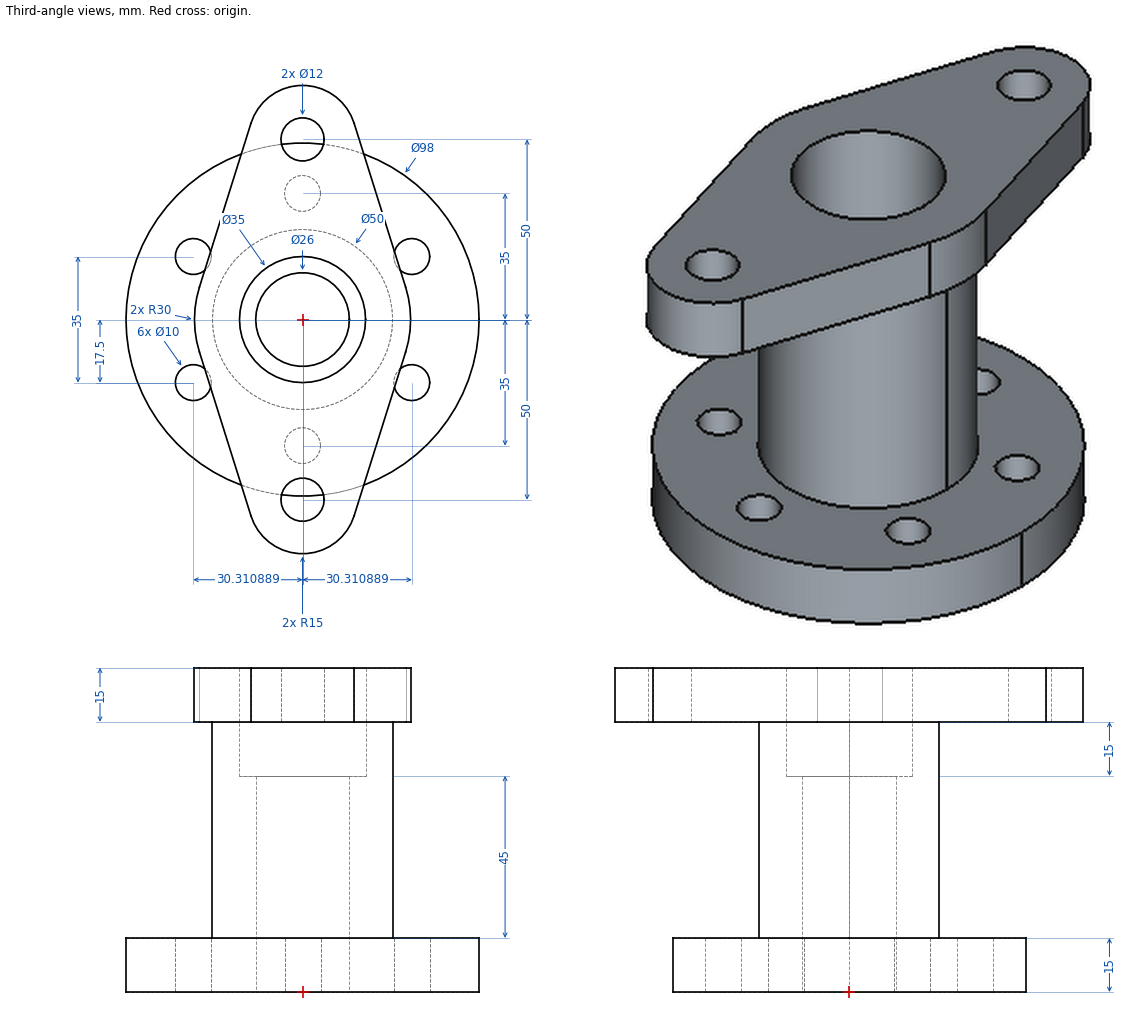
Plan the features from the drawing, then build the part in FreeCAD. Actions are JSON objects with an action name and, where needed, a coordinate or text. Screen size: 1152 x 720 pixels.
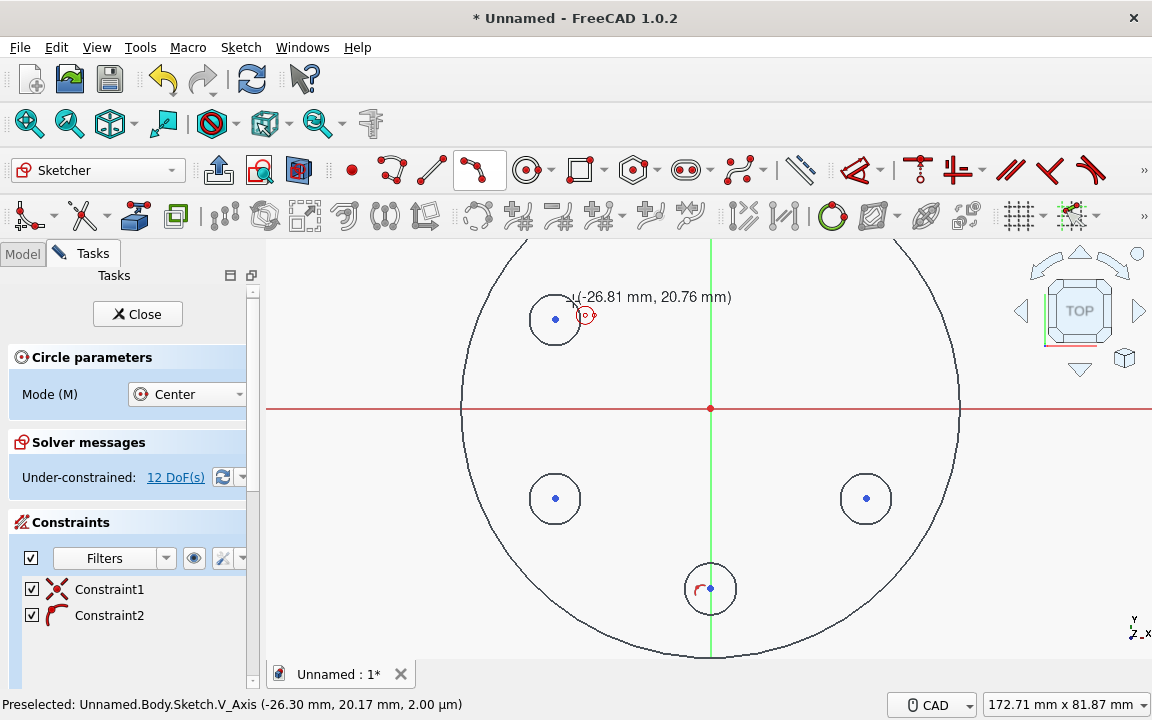
{"action": "left_click", "coordinate": [711, 409]}
{"action": "left_click", "coordinate": [758, 361]}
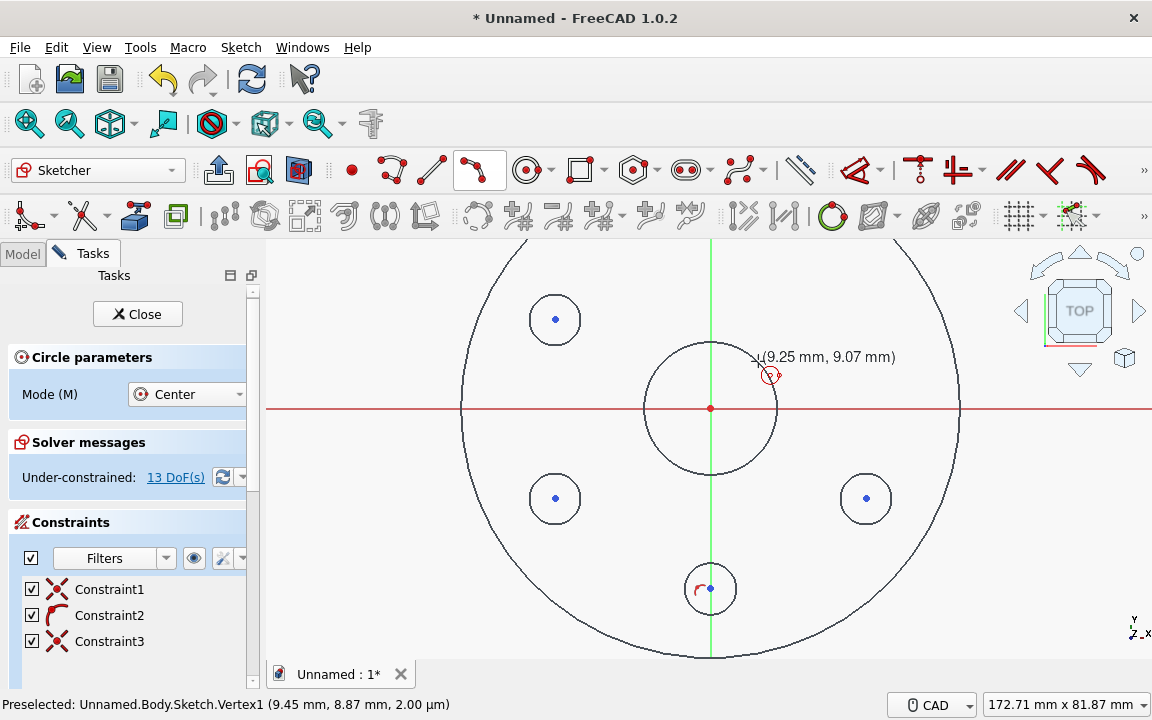
{"action": "left_click", "coordinate": [866, 319]}
{"action": "left_click", "coordinate": [884, 301]}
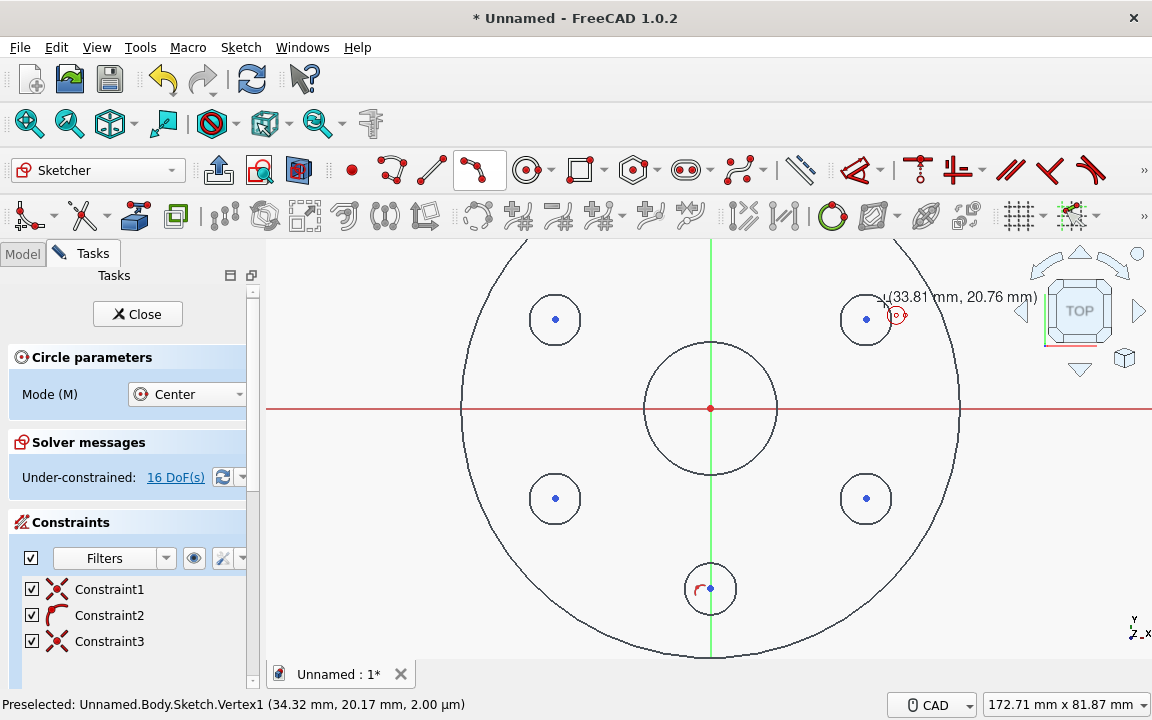
{"action": "scroll", "coordinate": [555, 498], "scroll_direction": "down", "scroll_amount": 3}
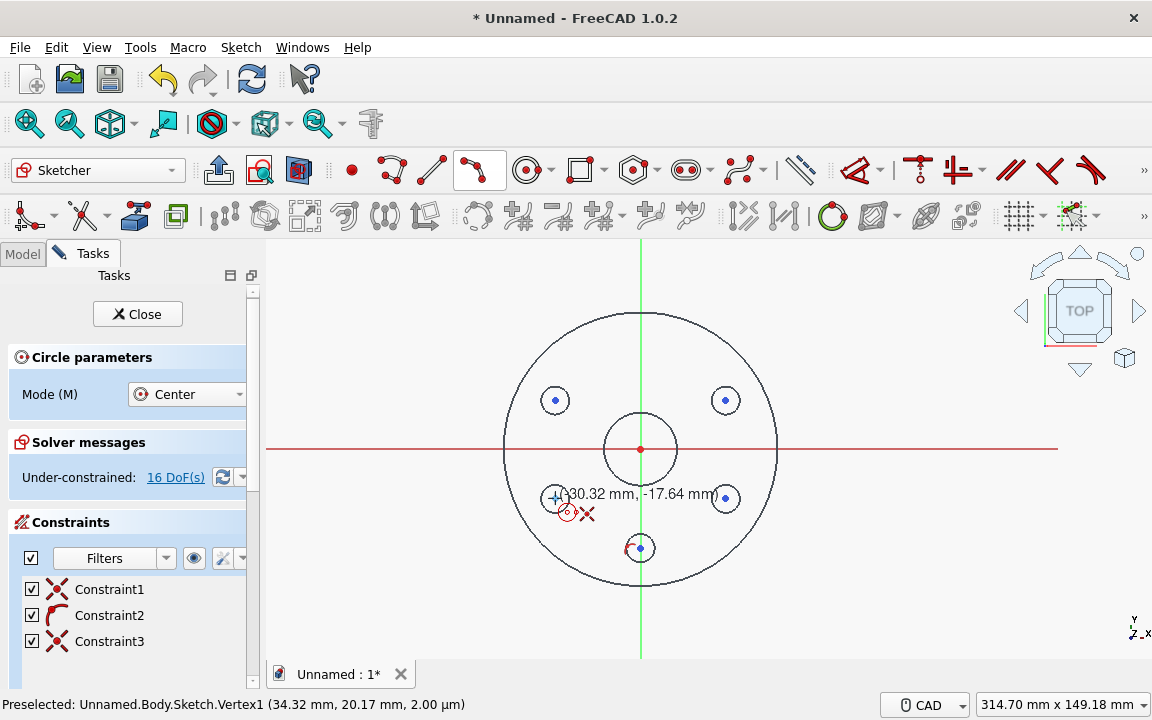
{"action": "scroll", "coordinate": [641, 351], "scroll_direction": "up", "scroll_amount": 3}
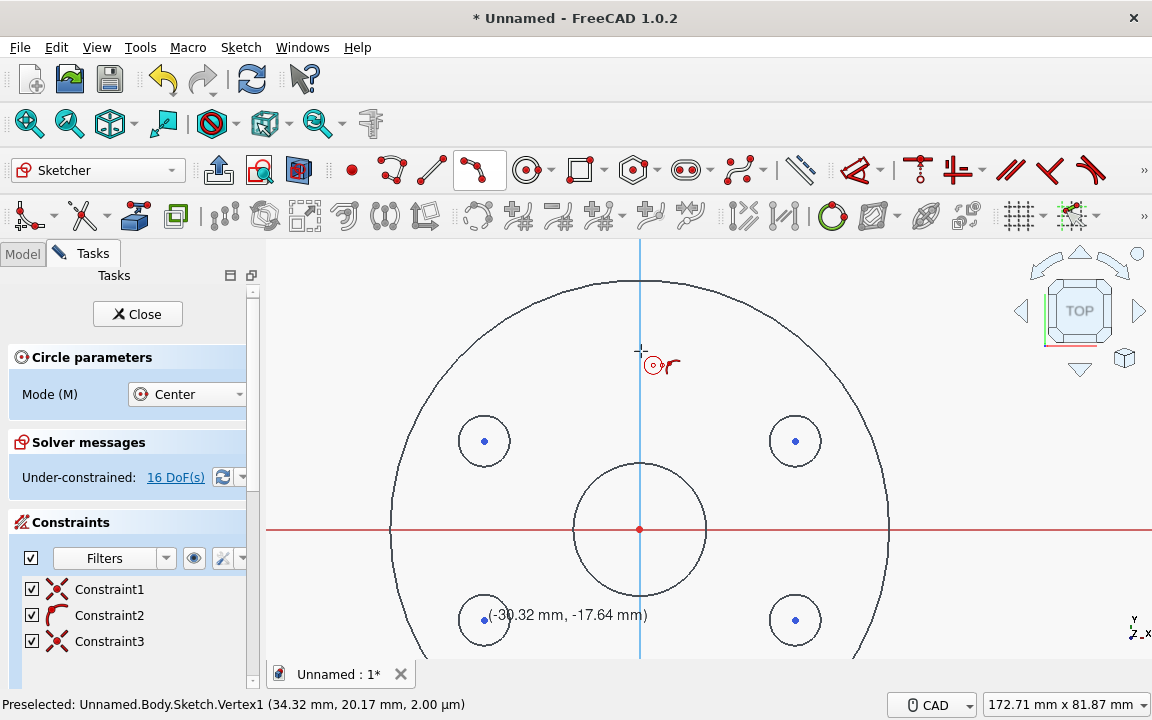
{"action": "left_click", "coordinate": [640, 350]}
{"action": "left_click", "coordinate": [658, 332]}
{"action": "key", "text": "Escape"}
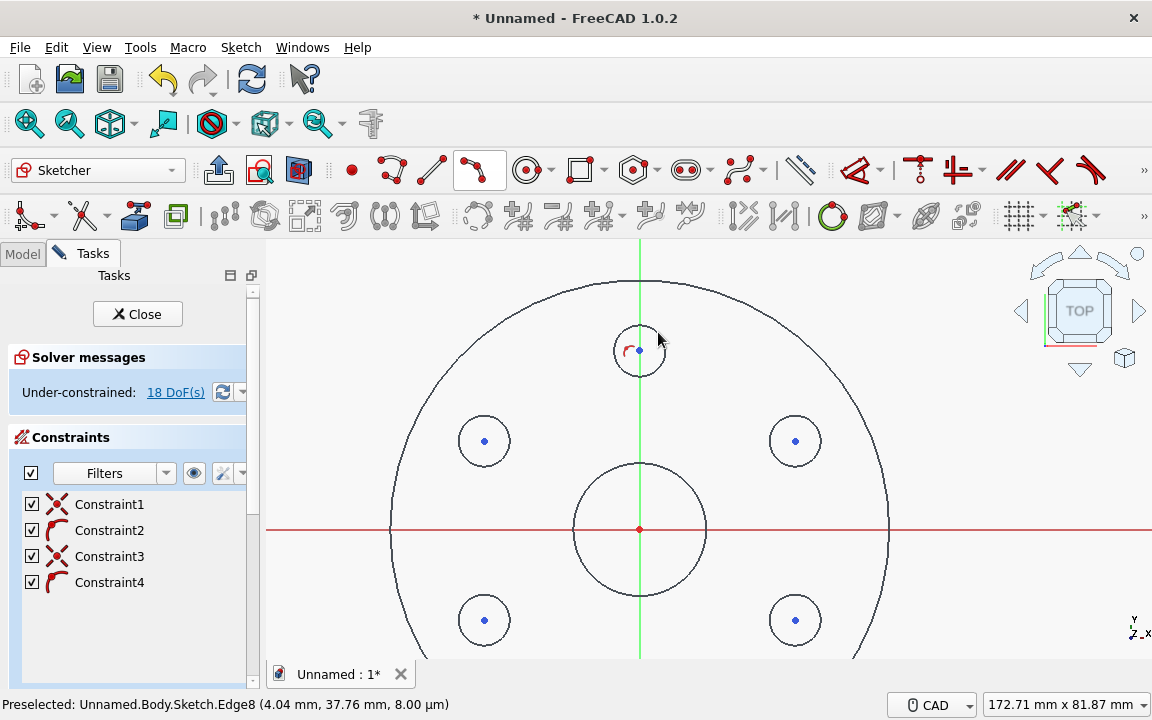
{"action": "left_click", "coordinate": [502, 602]}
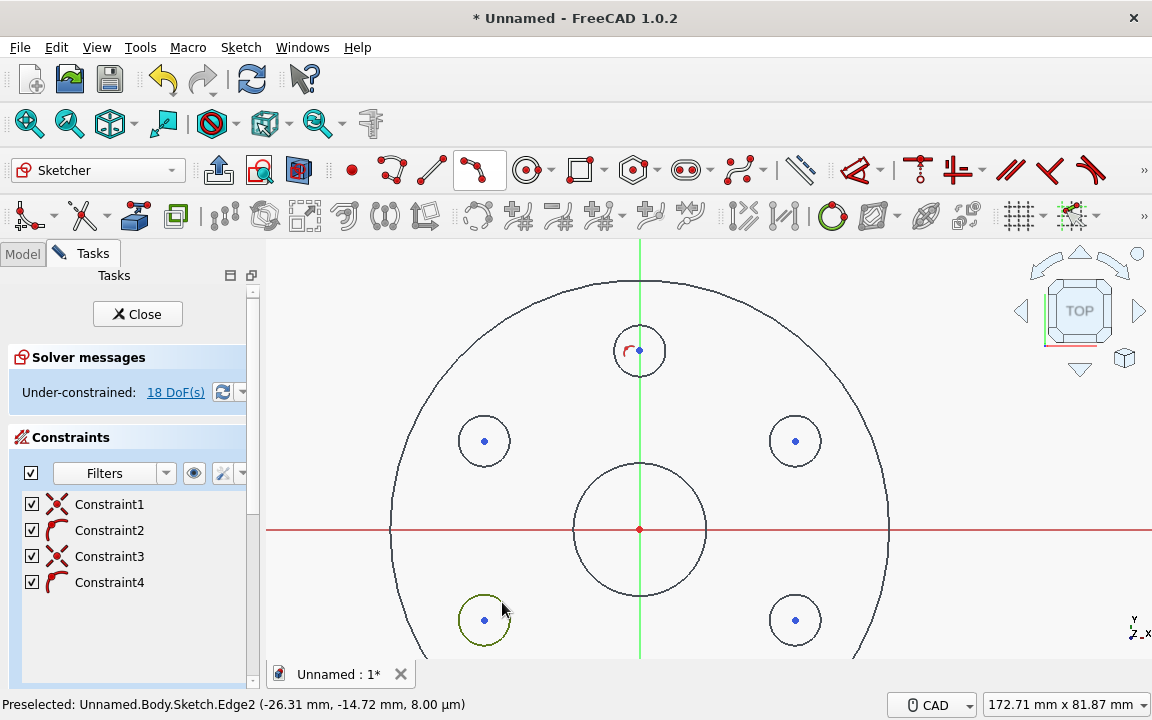
{"action": "scroll", "coordinate": [641, 351], "scroll_direction": "down", "scroll_amount": 3}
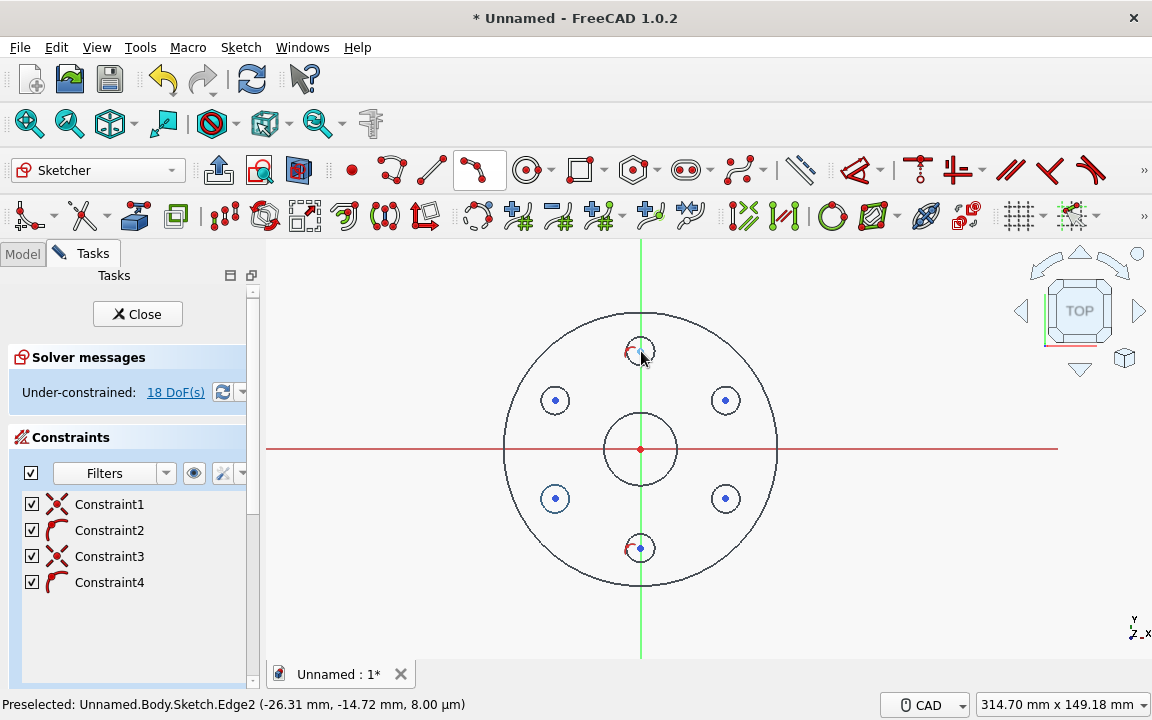
{"action": "scroll", "coordinate": [650, 538], "scroll_direction": "up", "scroll_amount": 2}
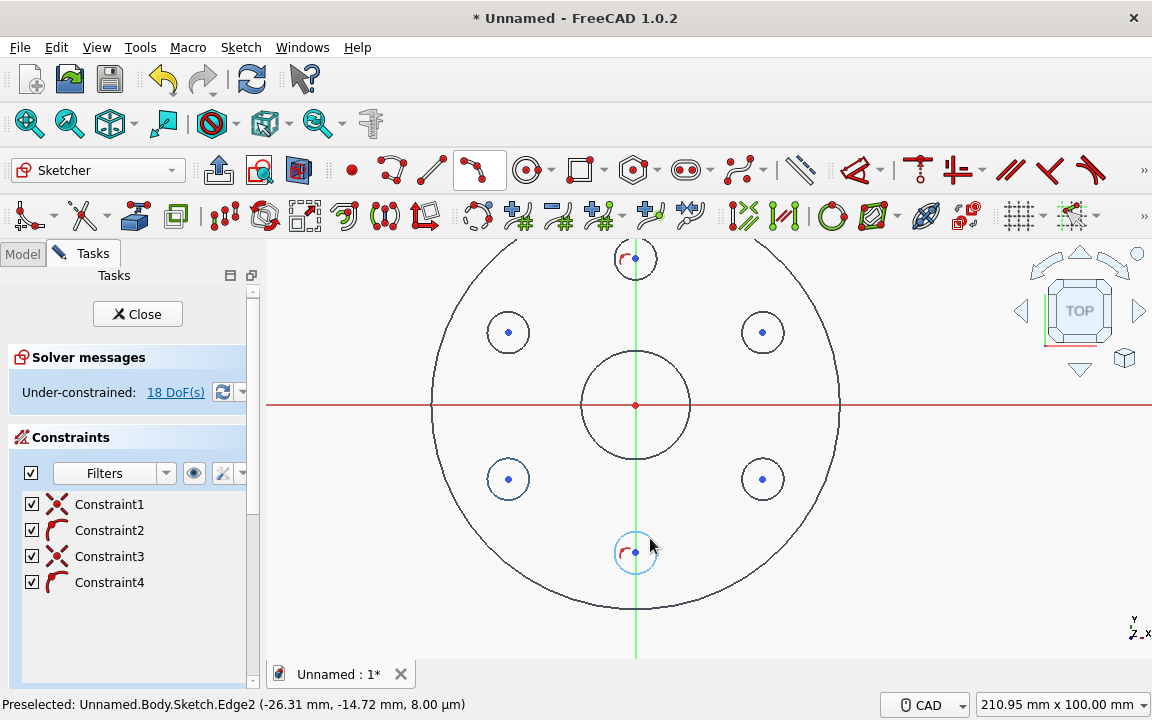
{"action": "left_click", "coordinate": [651, 538]}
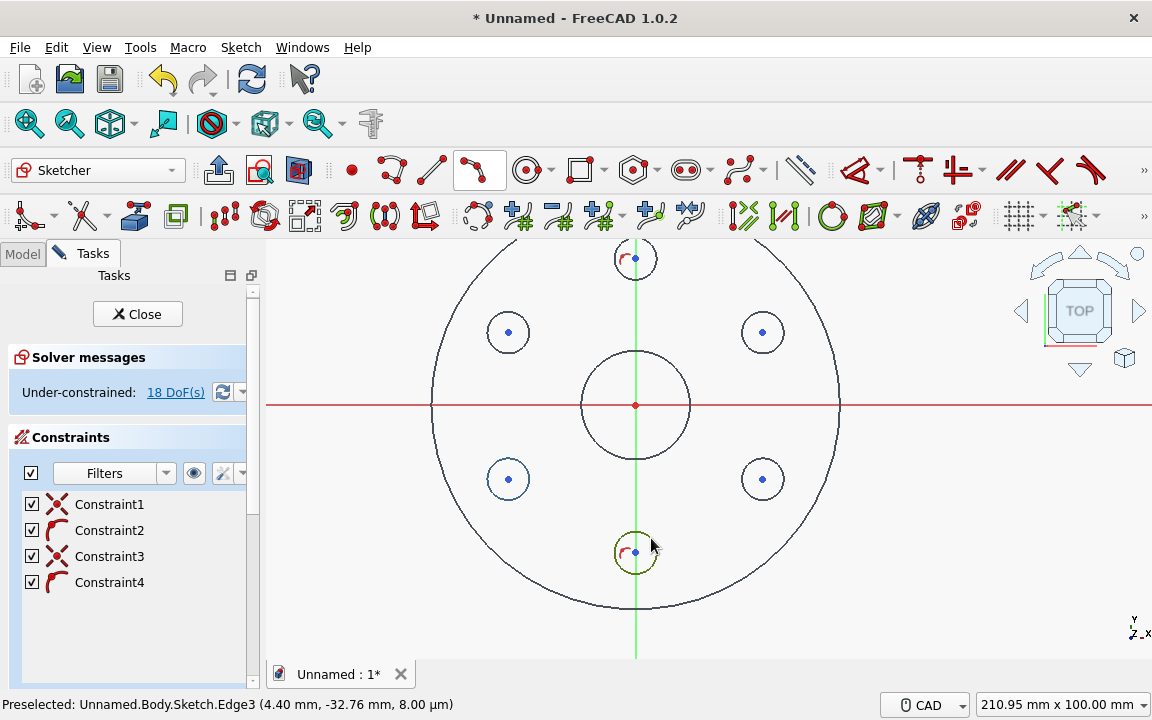
{"action": "left_click", "coordinate": [778, 464]}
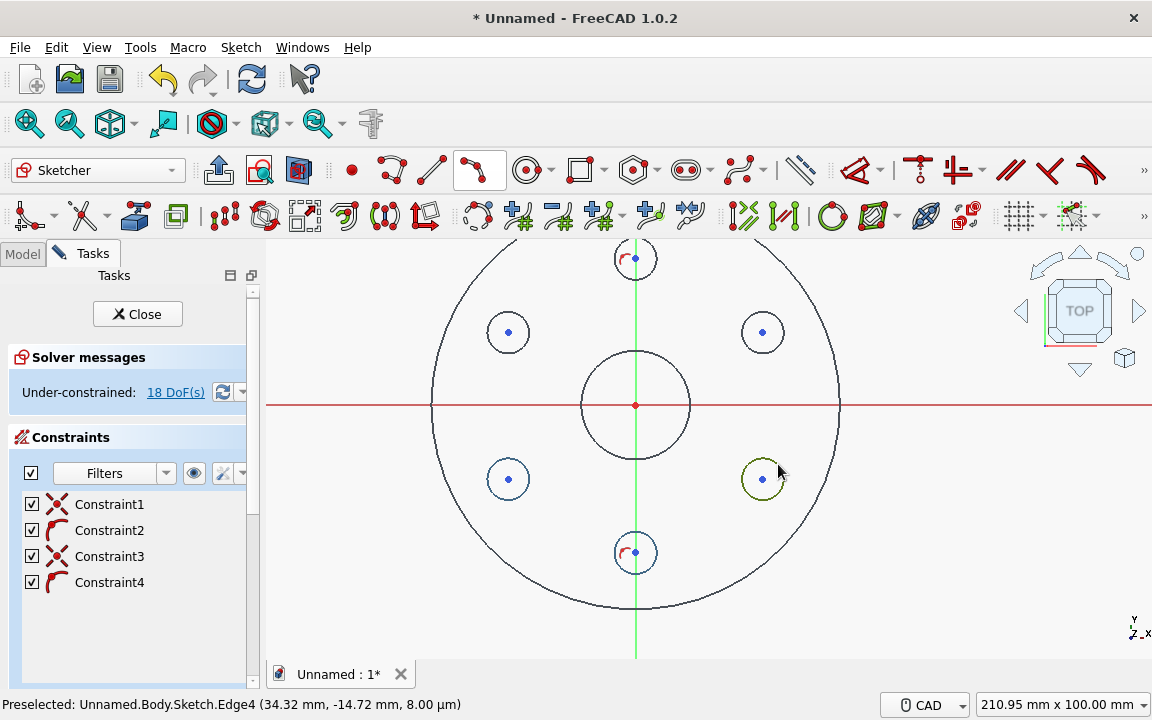
{"action": "left_click", "coordinate": [523, 318]}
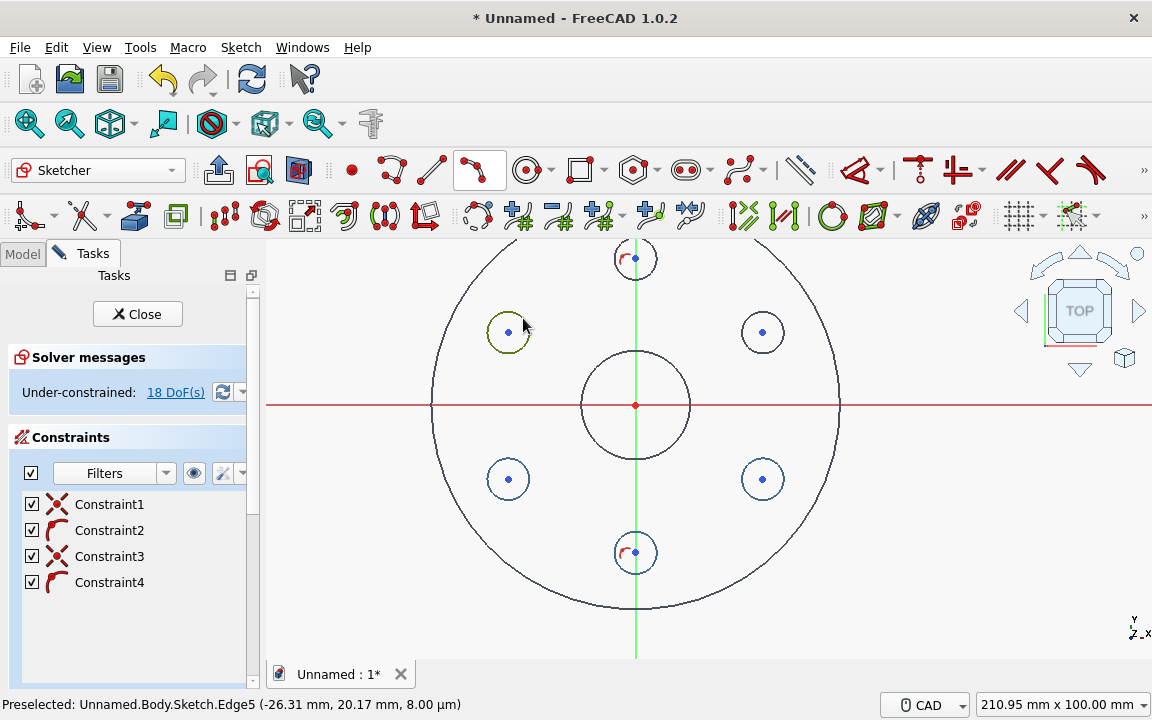
{"action": "left_click", "coordinate": [778, 318]}